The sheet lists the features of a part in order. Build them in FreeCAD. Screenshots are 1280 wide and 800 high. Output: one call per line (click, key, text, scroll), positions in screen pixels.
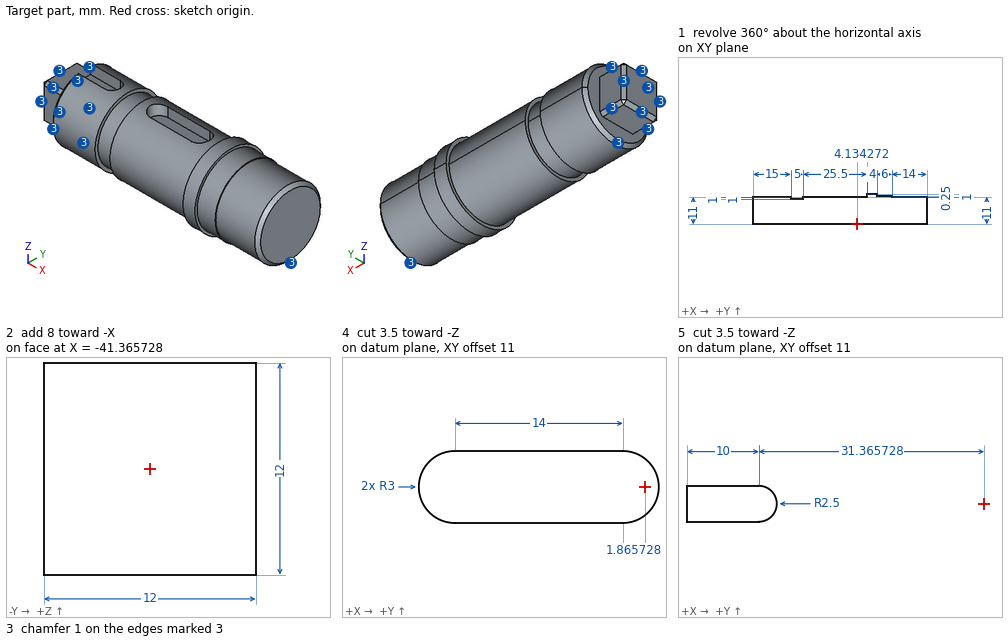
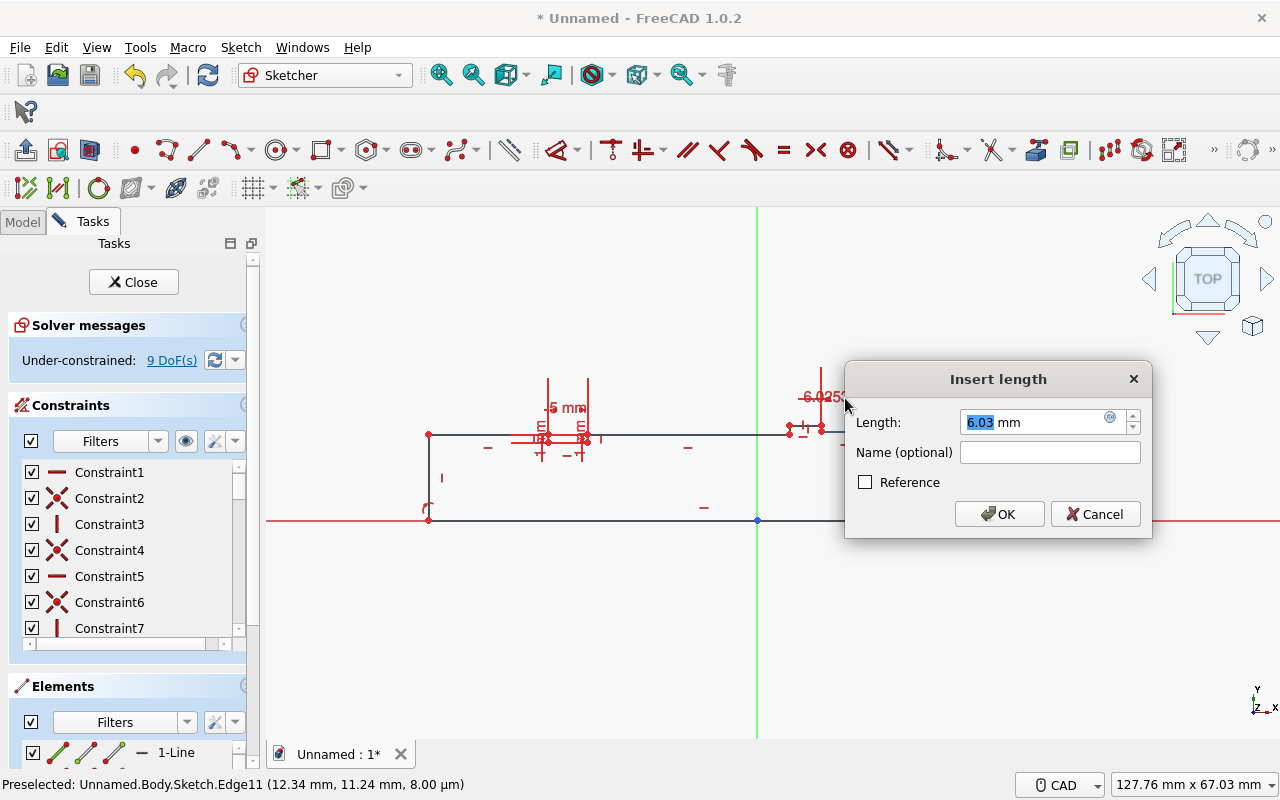
text(6)
key(Return)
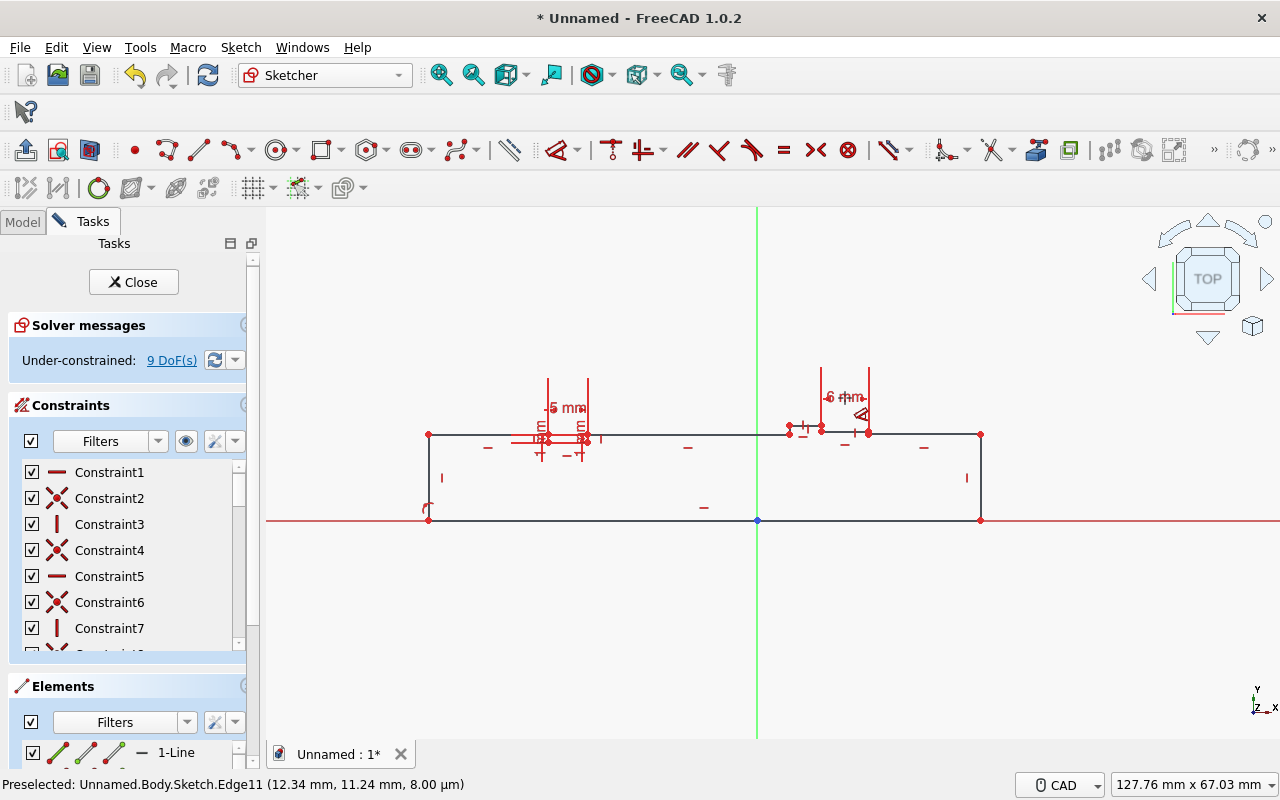
scroll(812, 426, up, 2)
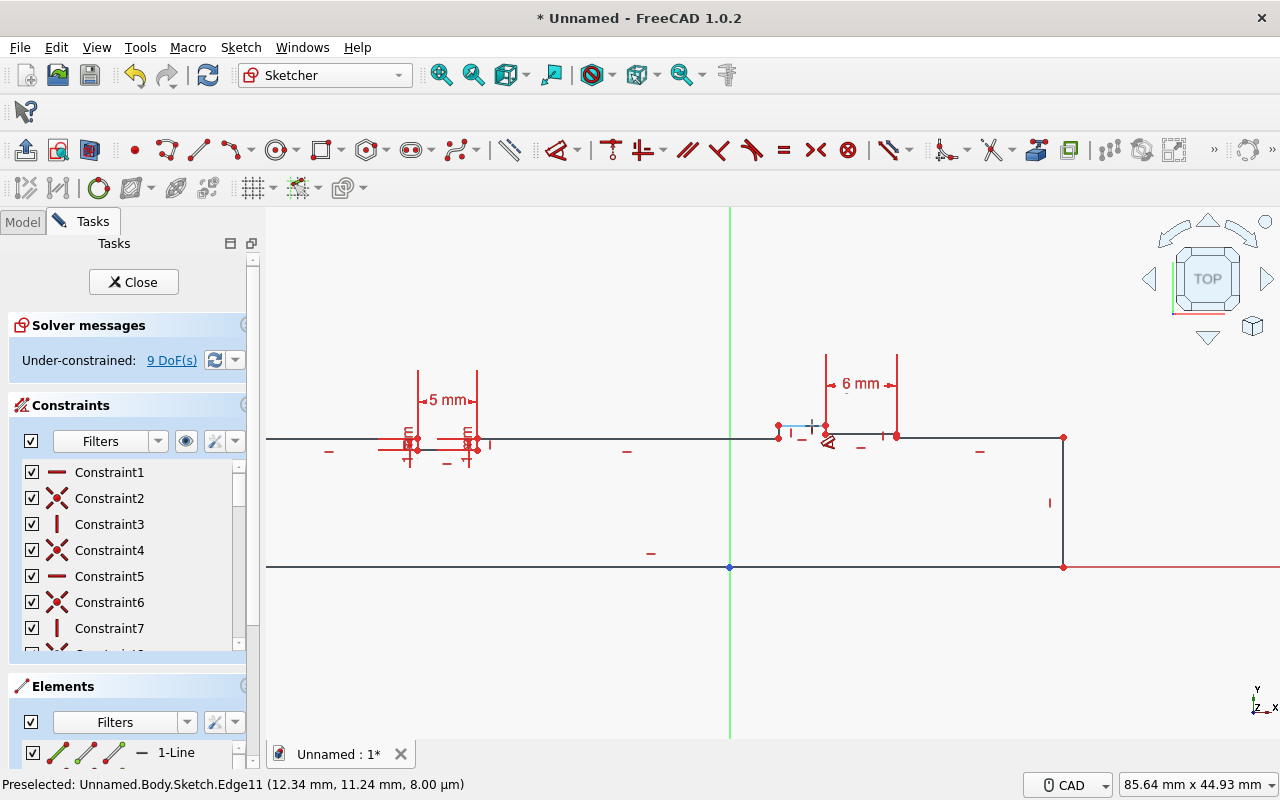
click(811, 426)
click(791, 392)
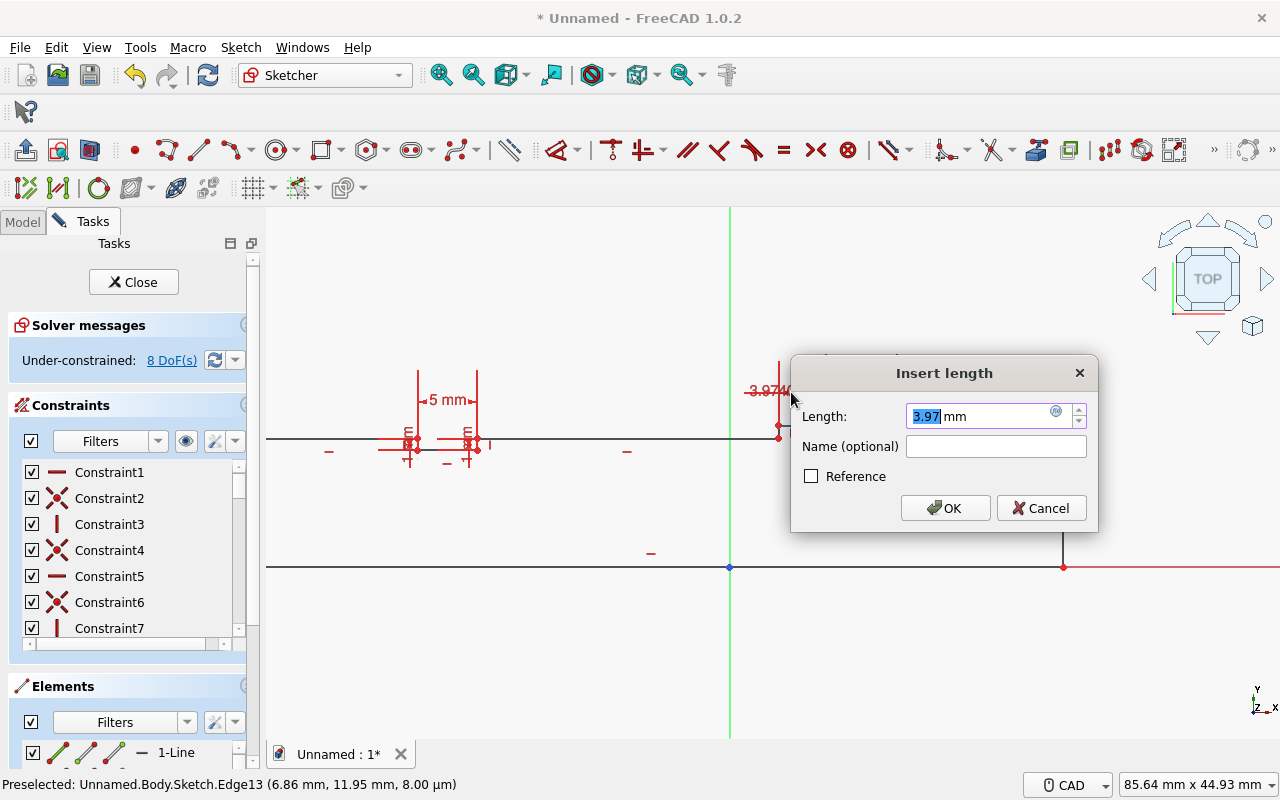
text(4)
key(Return)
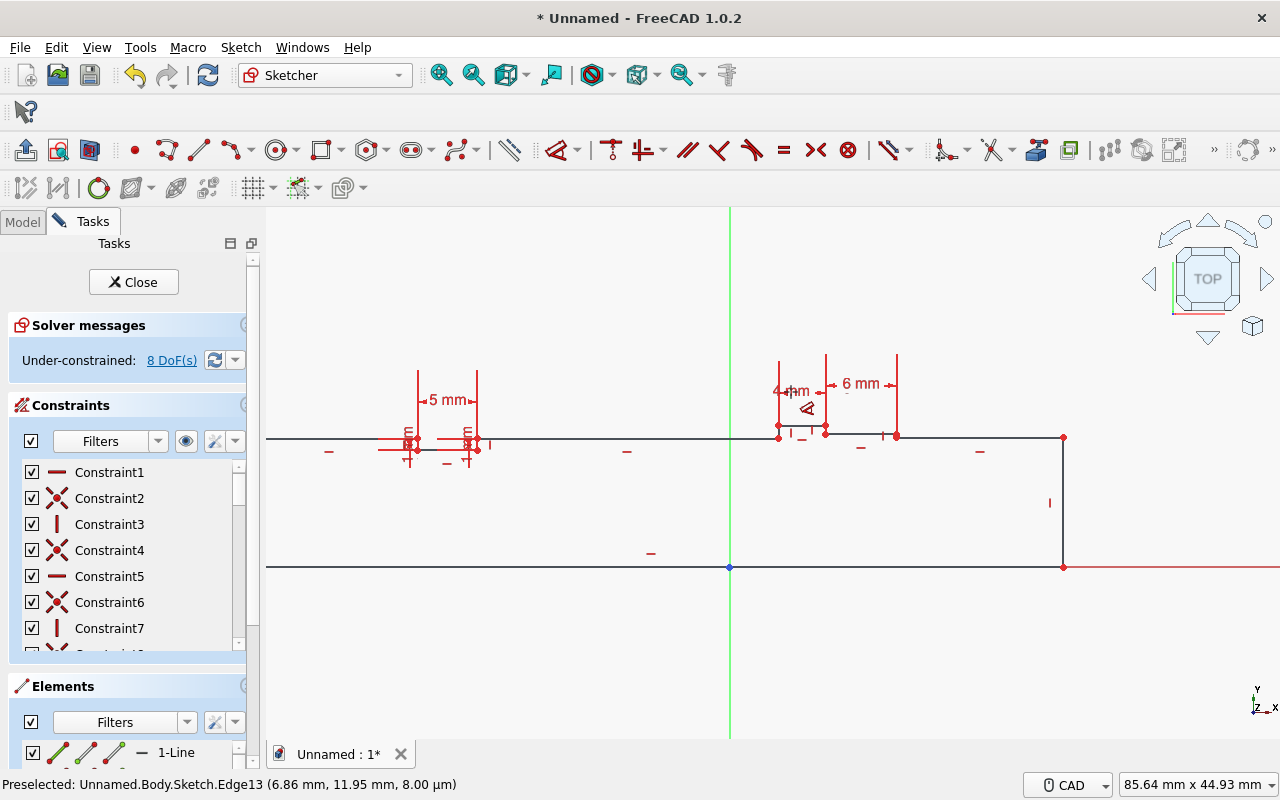
scroll(779, 432, up, 7)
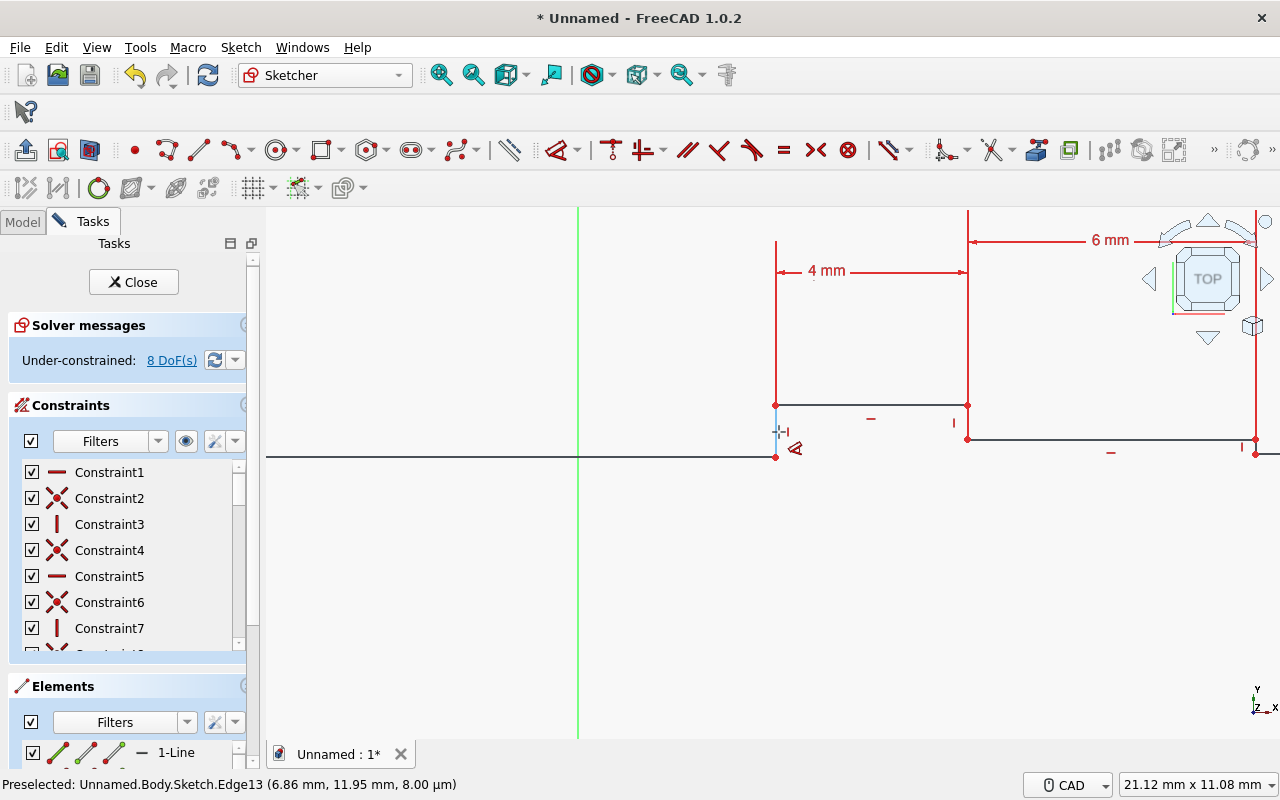
click(776, 431)
click(810, 431)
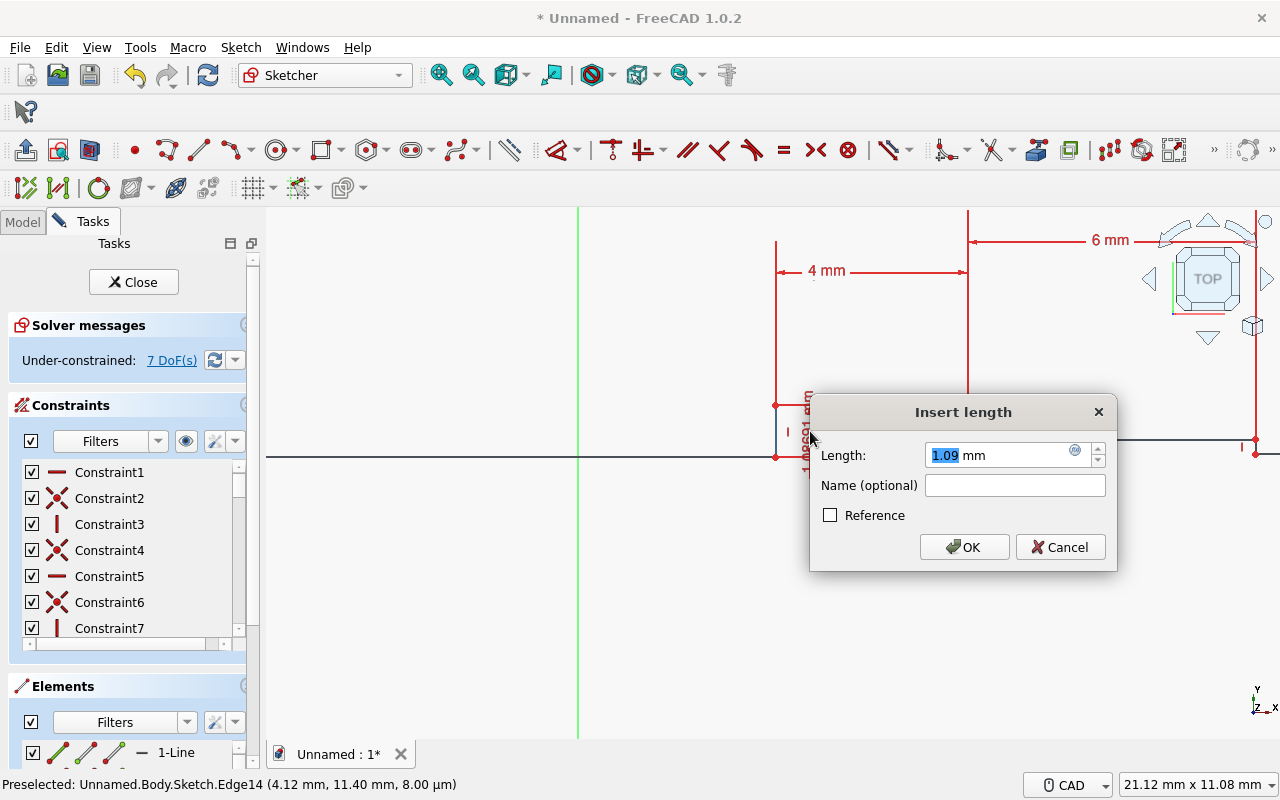
text(1)
key(Return)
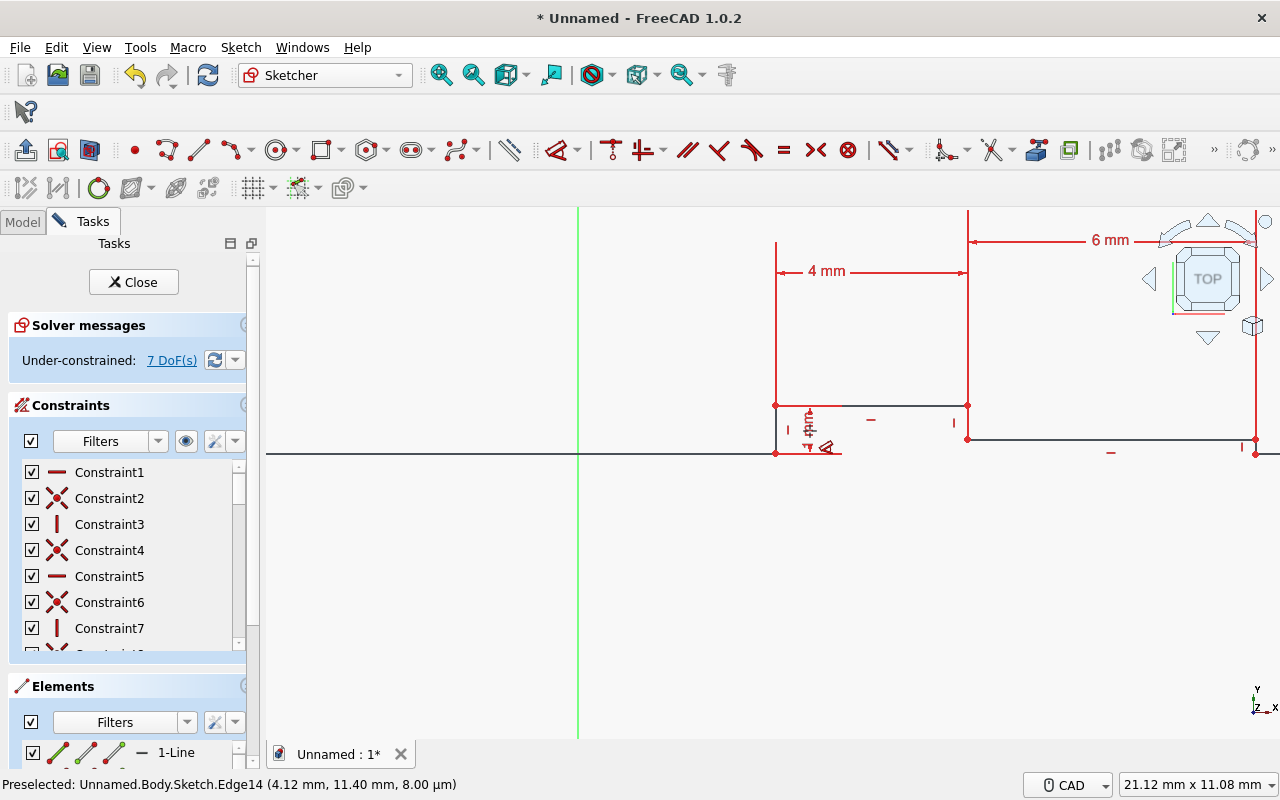
scroll(792, 430, down, 9)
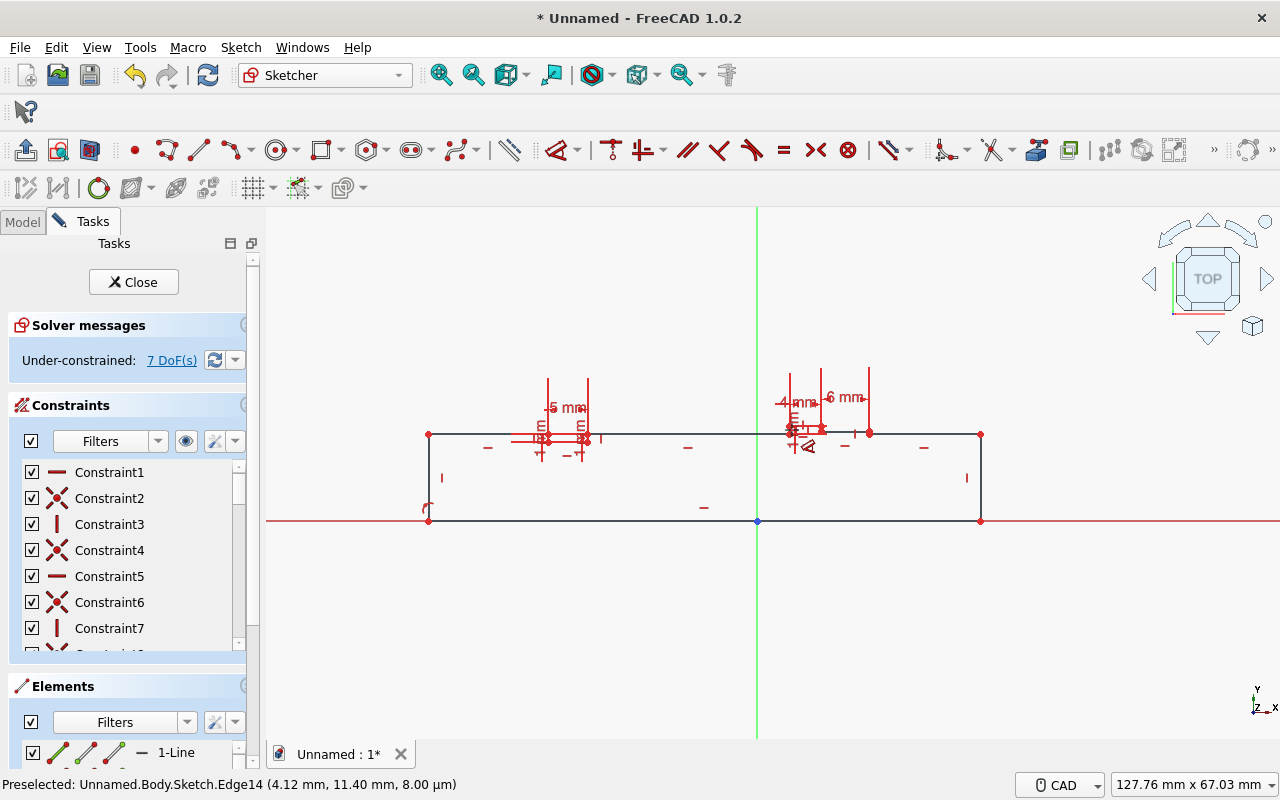
click(512, 434)
click(488, 400)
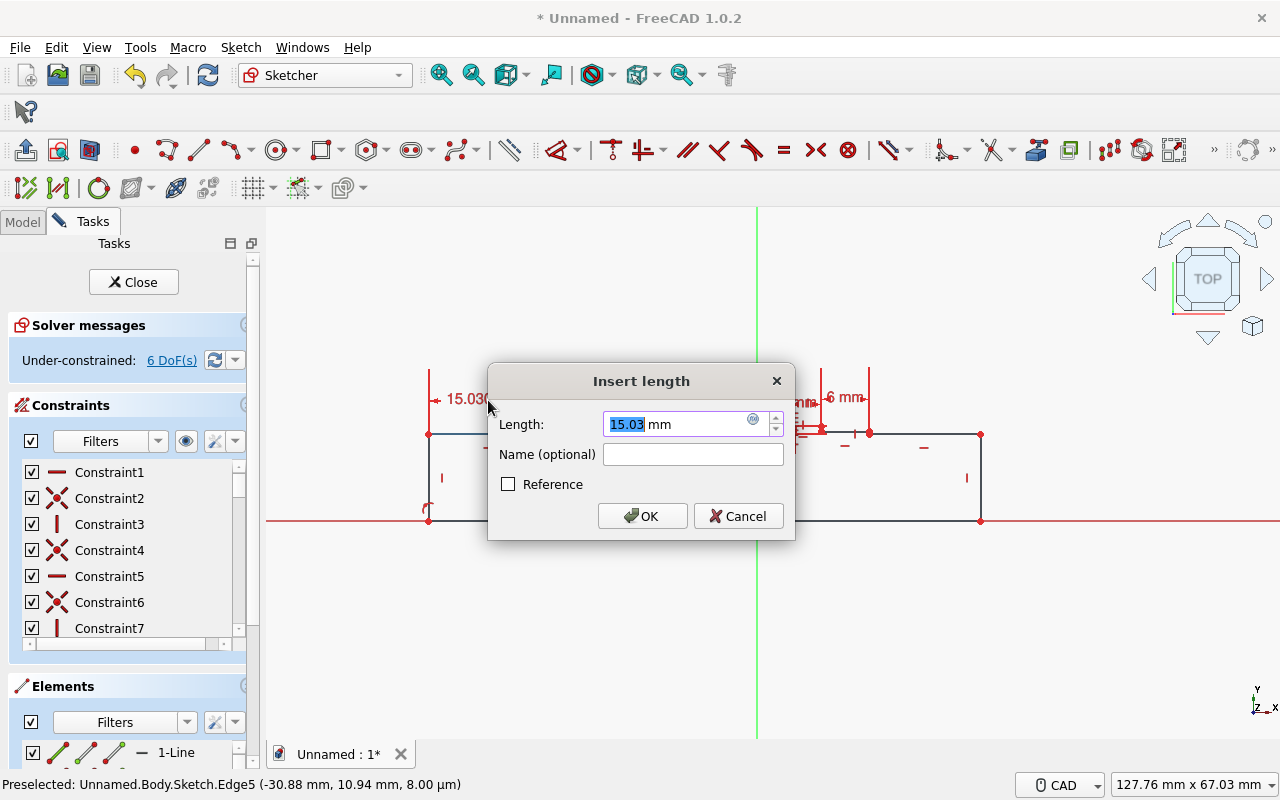
text(15)
key(Return)